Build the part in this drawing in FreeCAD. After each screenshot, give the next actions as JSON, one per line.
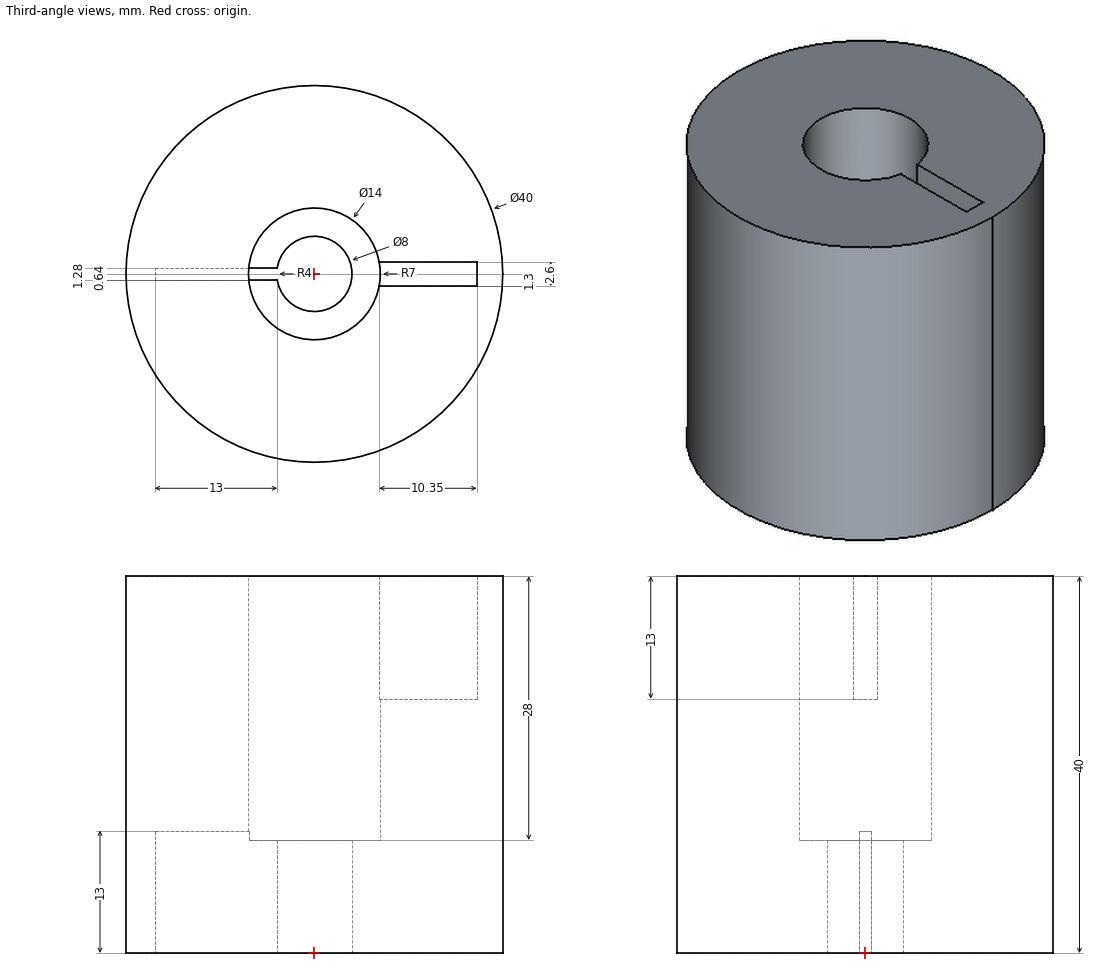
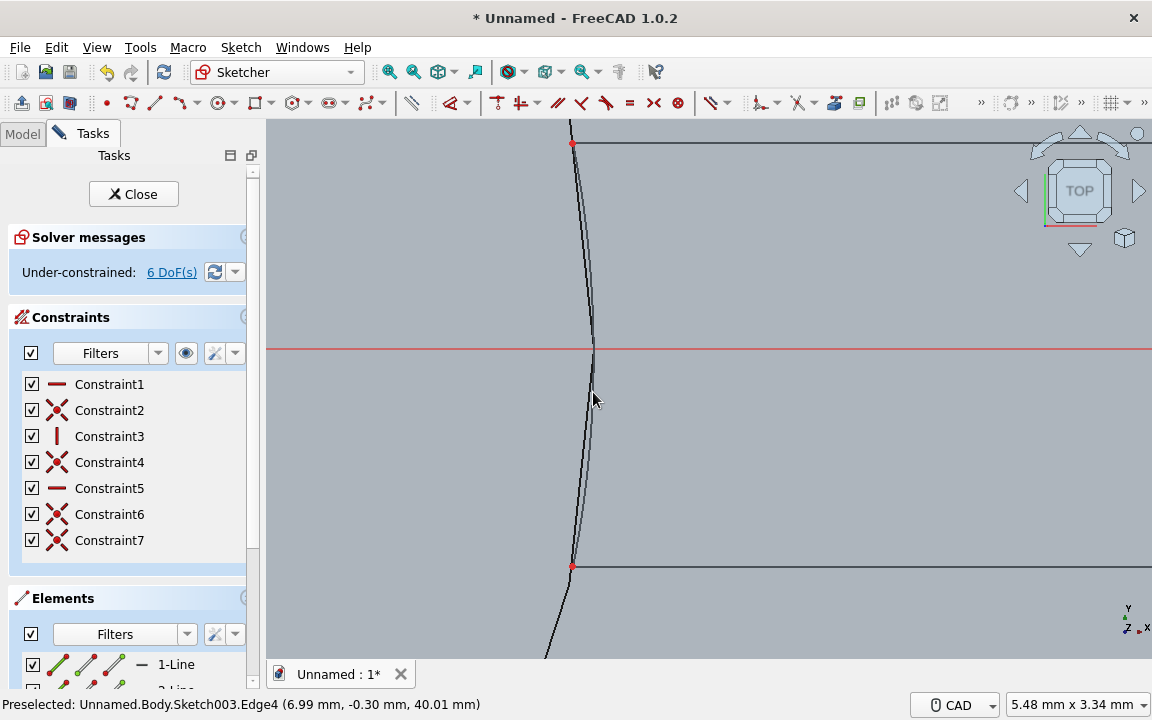
{"action": "scroll", "coordinate": [598, 397], "scroll_direction": "down", "scroll_amount": 9}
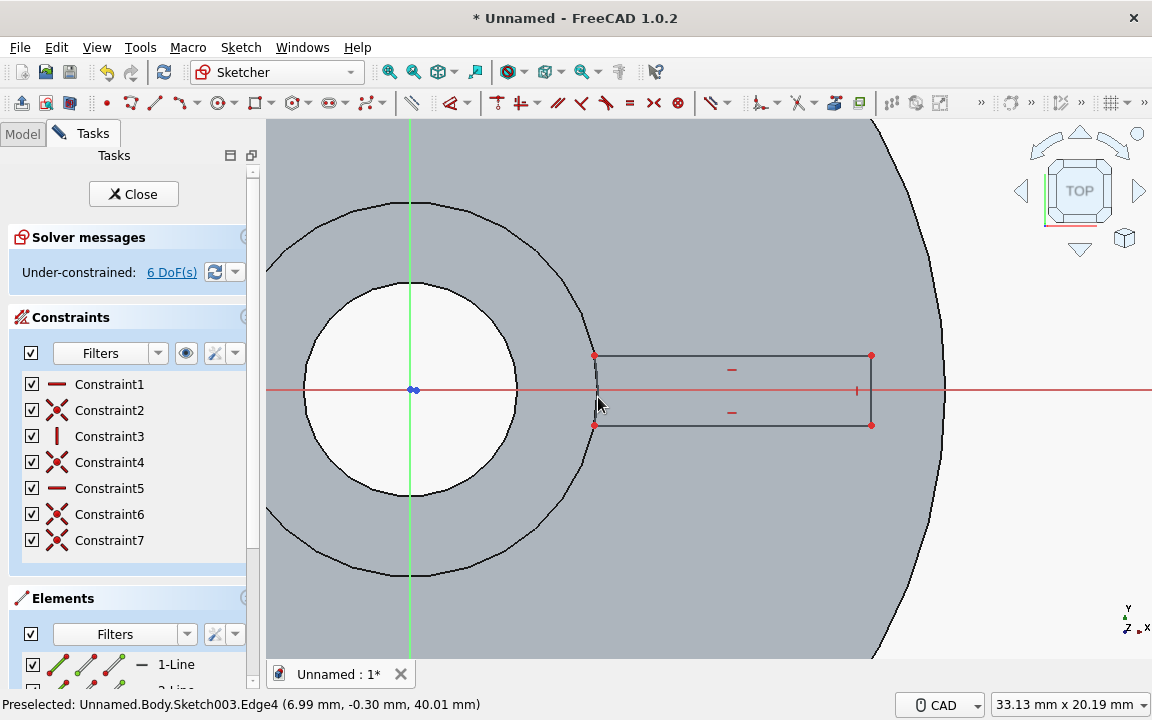
{"action": "left_click_drag", "start_coordinate": [400, 380], "coordinate": [427, 401]}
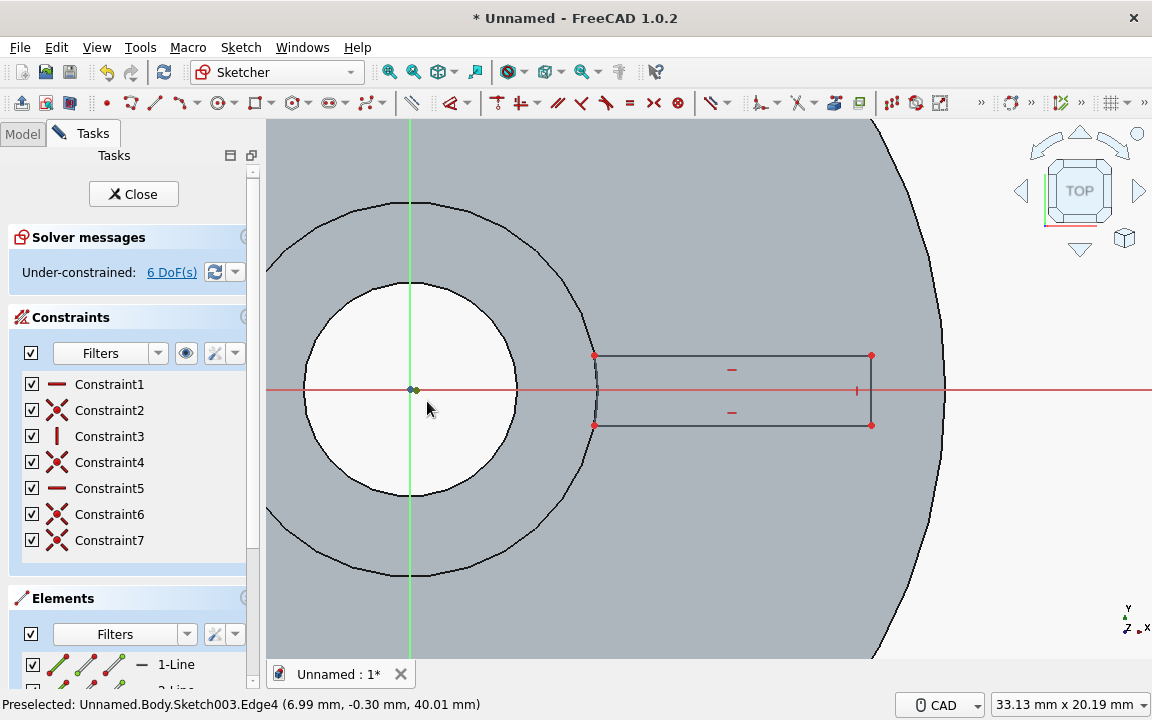
{"action": "key", "text": "c"}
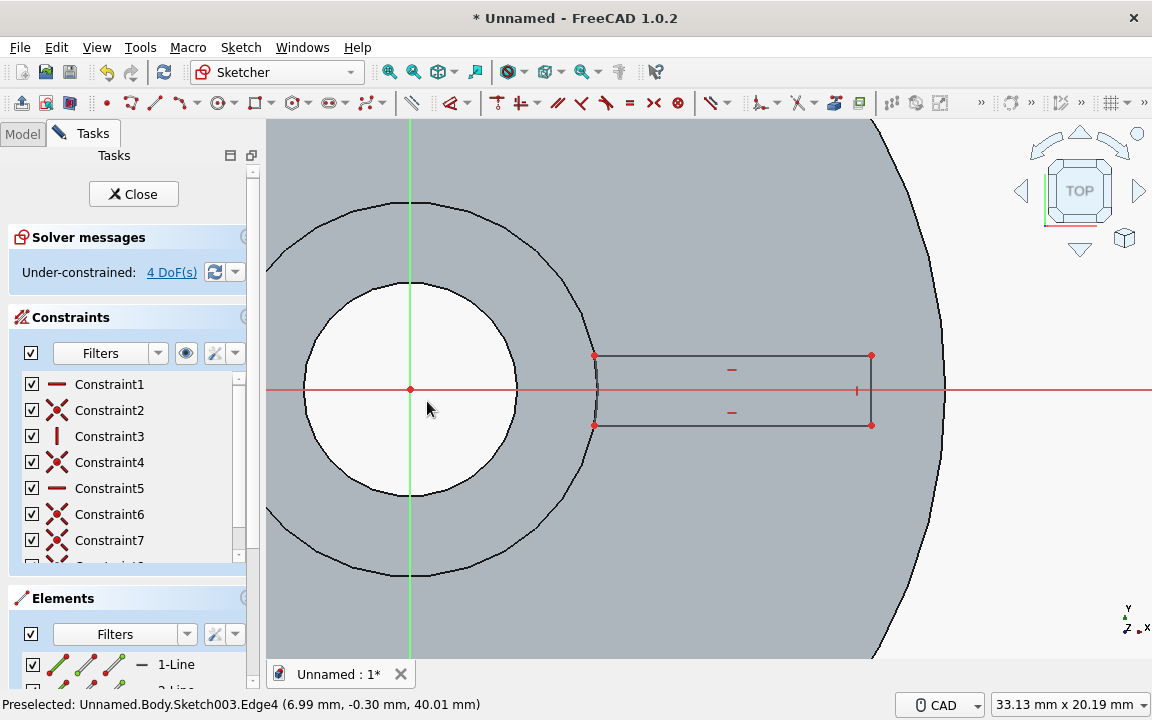
{"action": "left_click", "coordinate": [450, 104]}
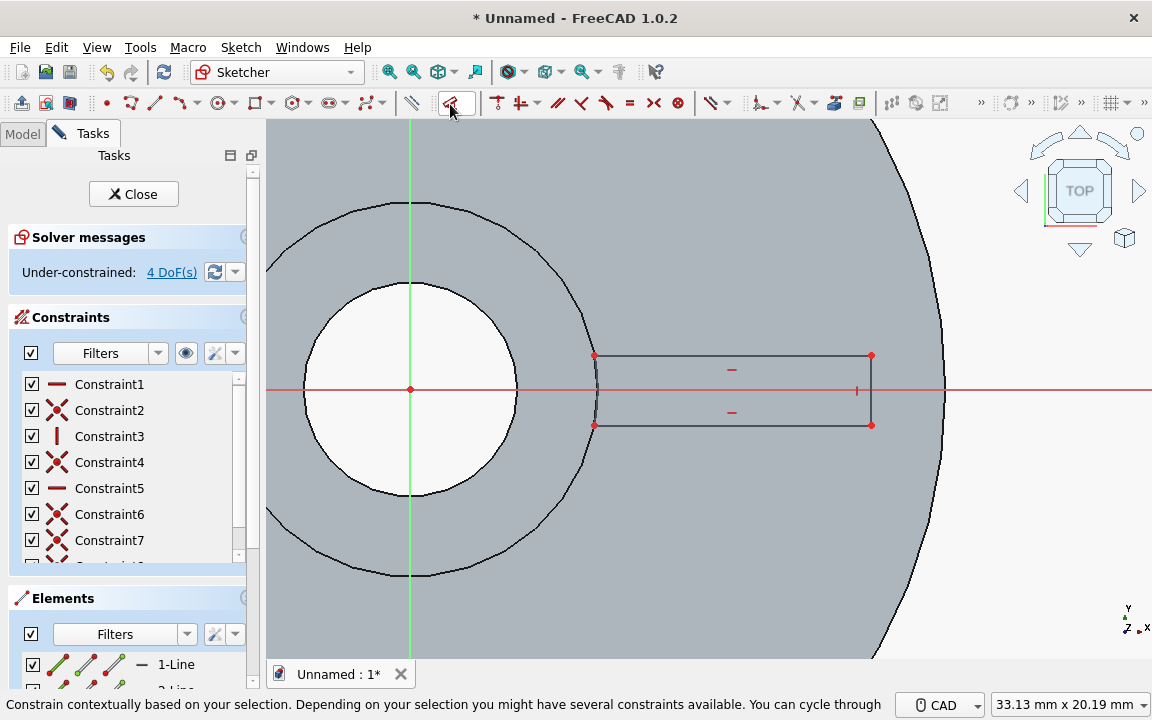
{"action": "left_click", "coordinate": [597, 405]}
{"action": "left_click", "coordinate": [629, 408]}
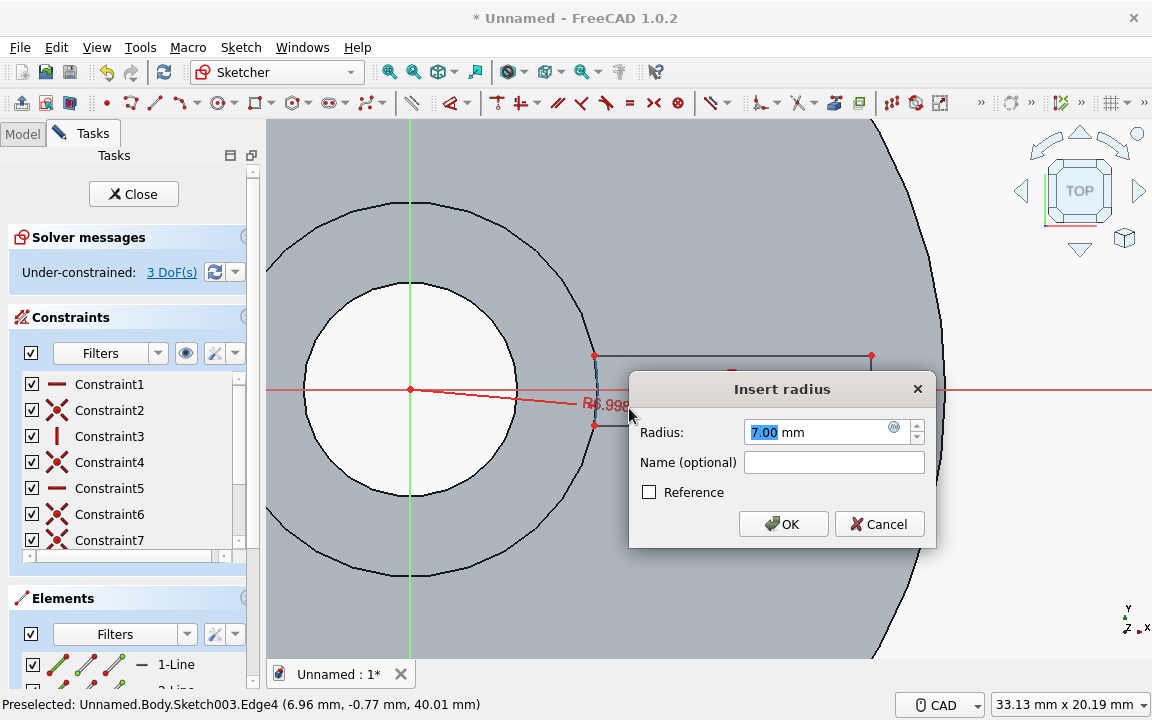
{"action": "type", "text": "7"}
{"action": "key", "text": "Return"}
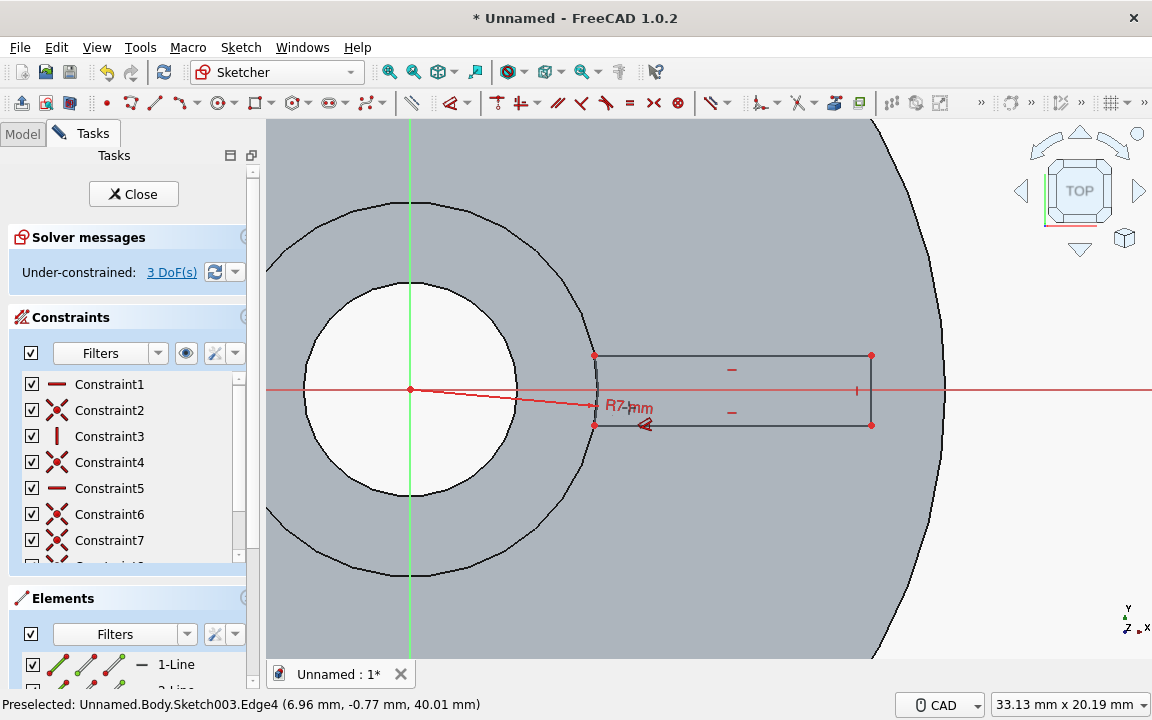
{"action": "left_click", "coordinate": [871, 405]}
{"action": "left_click", "coordinate": [905, 374]}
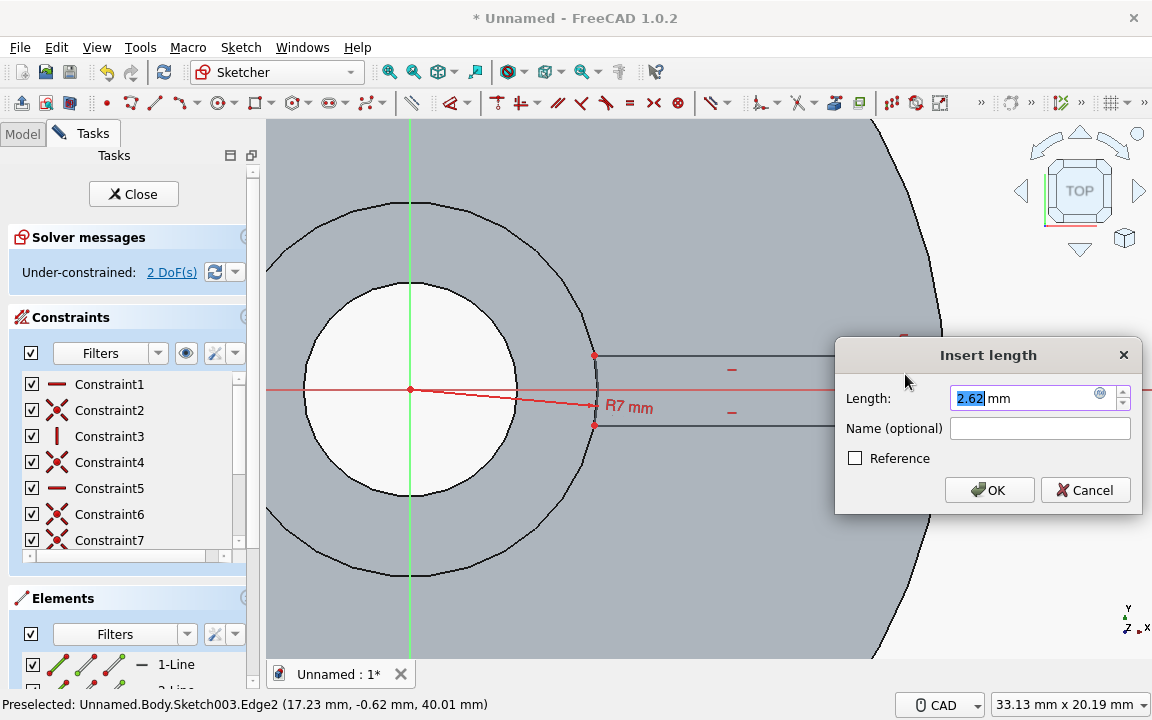
{"action": "type", "text": "2.6"}
{"action": "key", "text": "Return"}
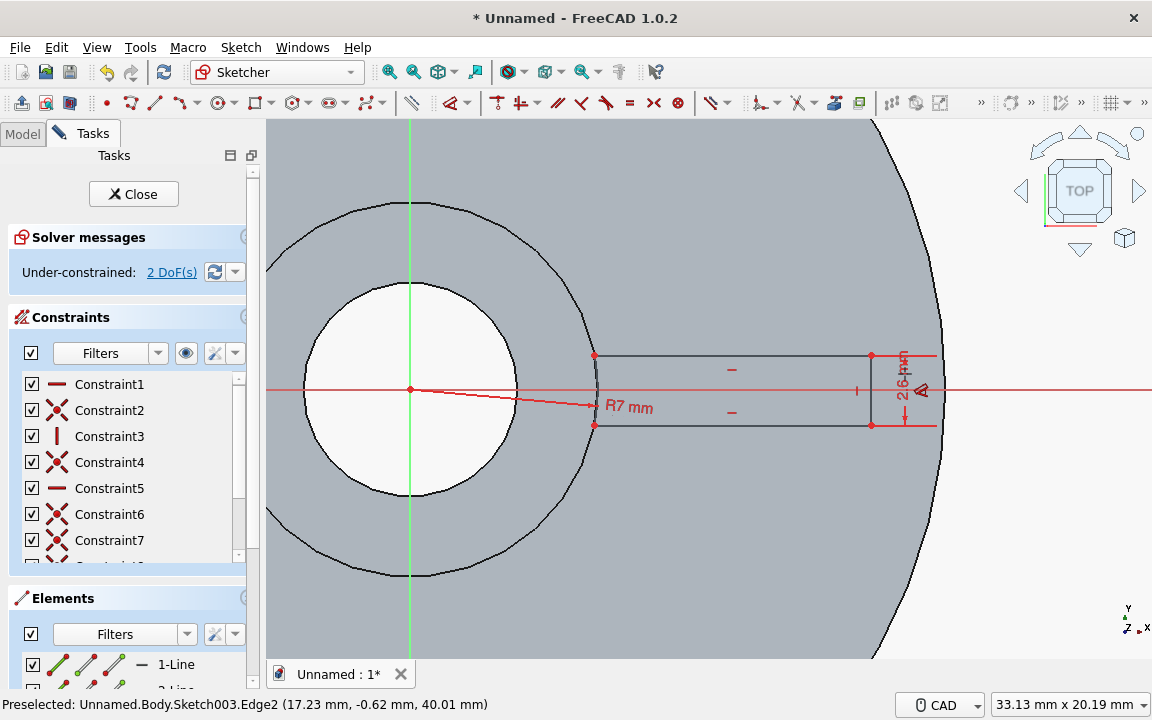
{"action": "left_click", "coordinate": [594, 426]}
{"action": "left_click", "coordinate": [376, 408]}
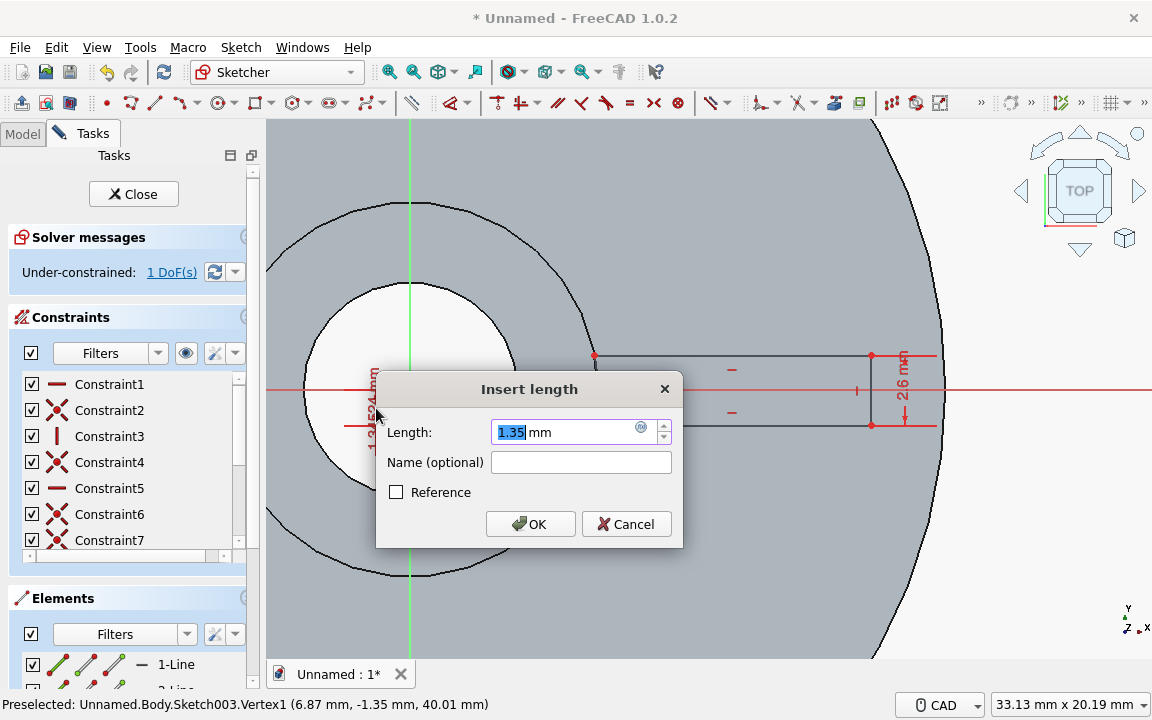
{"action": "type", "text": "1.3"}
{"action": "key", "text": "Return"}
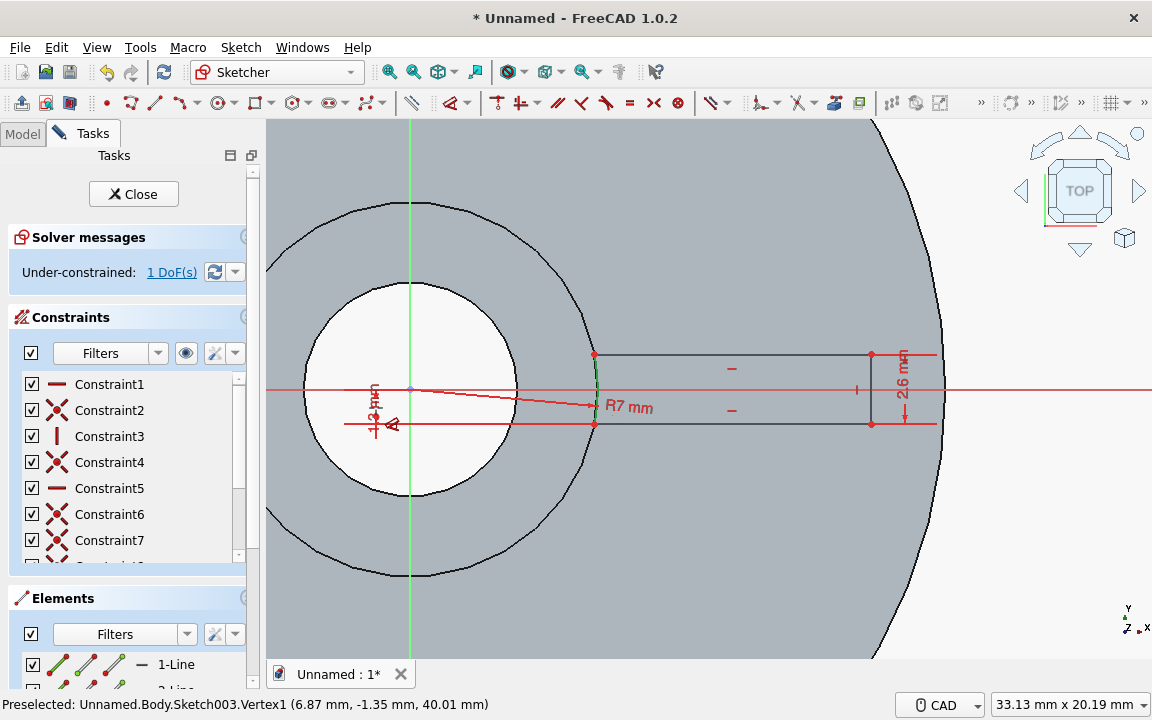
{"action": "left_click", "coordinate": [677, 424]}
{"action": "left_click", "coordinate": [733, 458]}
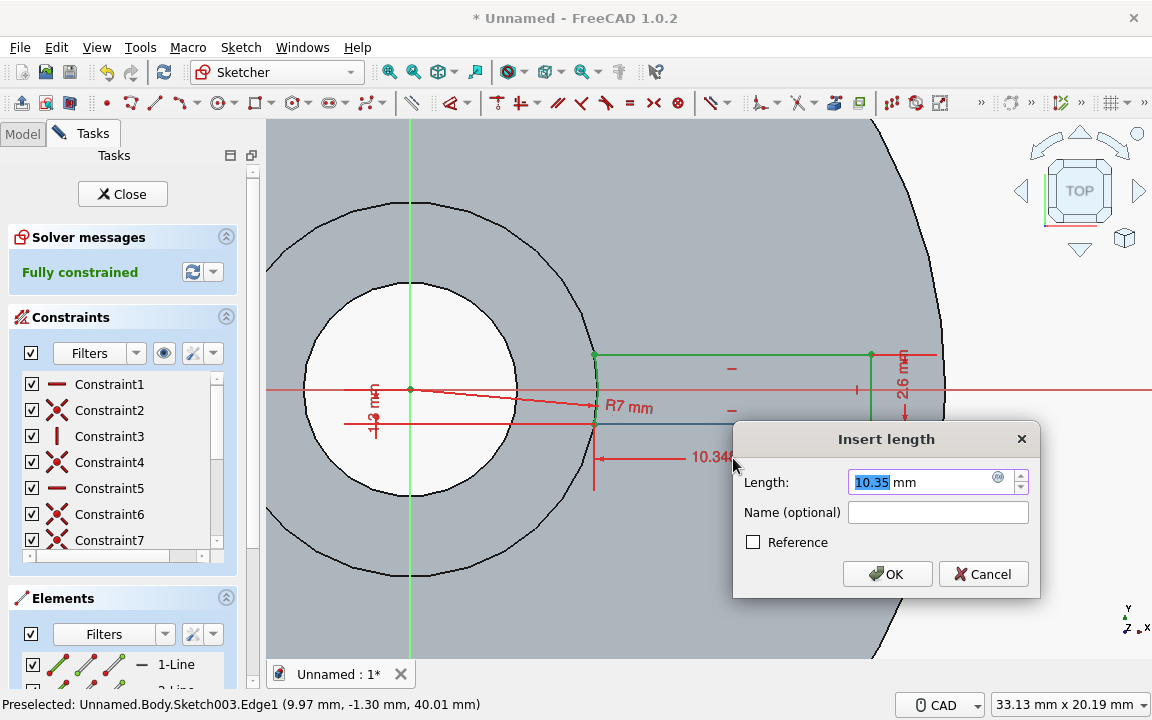
{"action": "type", "text": "10.35"}
{"action": "key", "text": "Return"}
{"action": "key", "text": "Escape"}